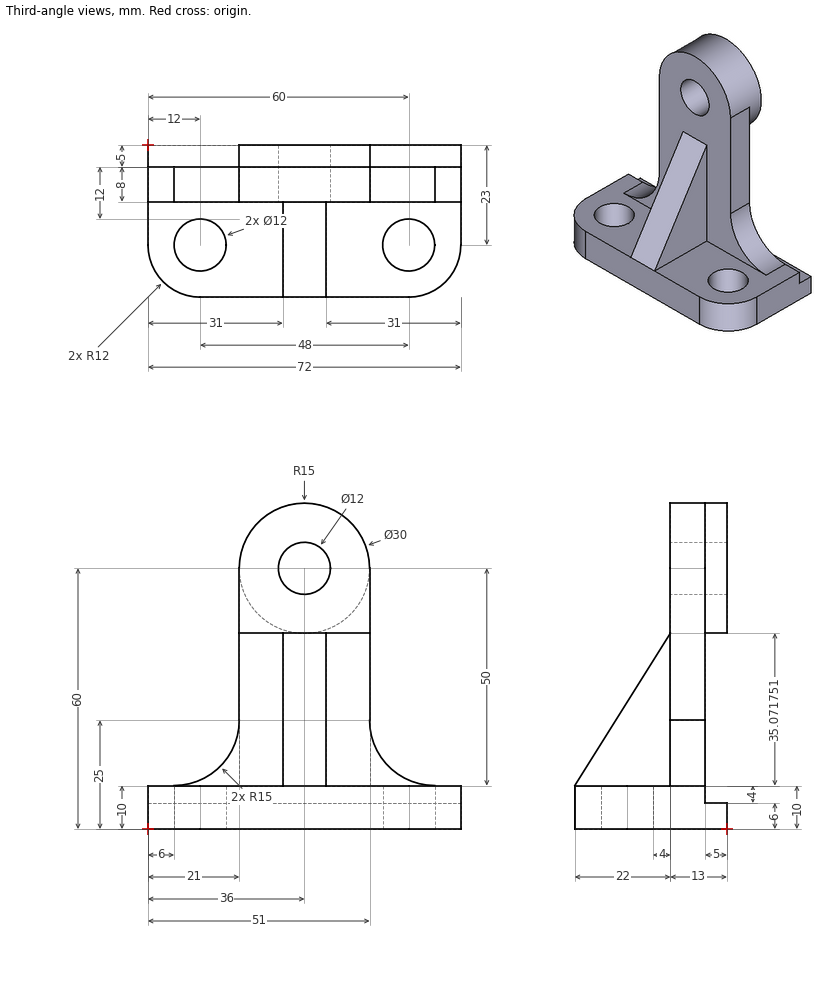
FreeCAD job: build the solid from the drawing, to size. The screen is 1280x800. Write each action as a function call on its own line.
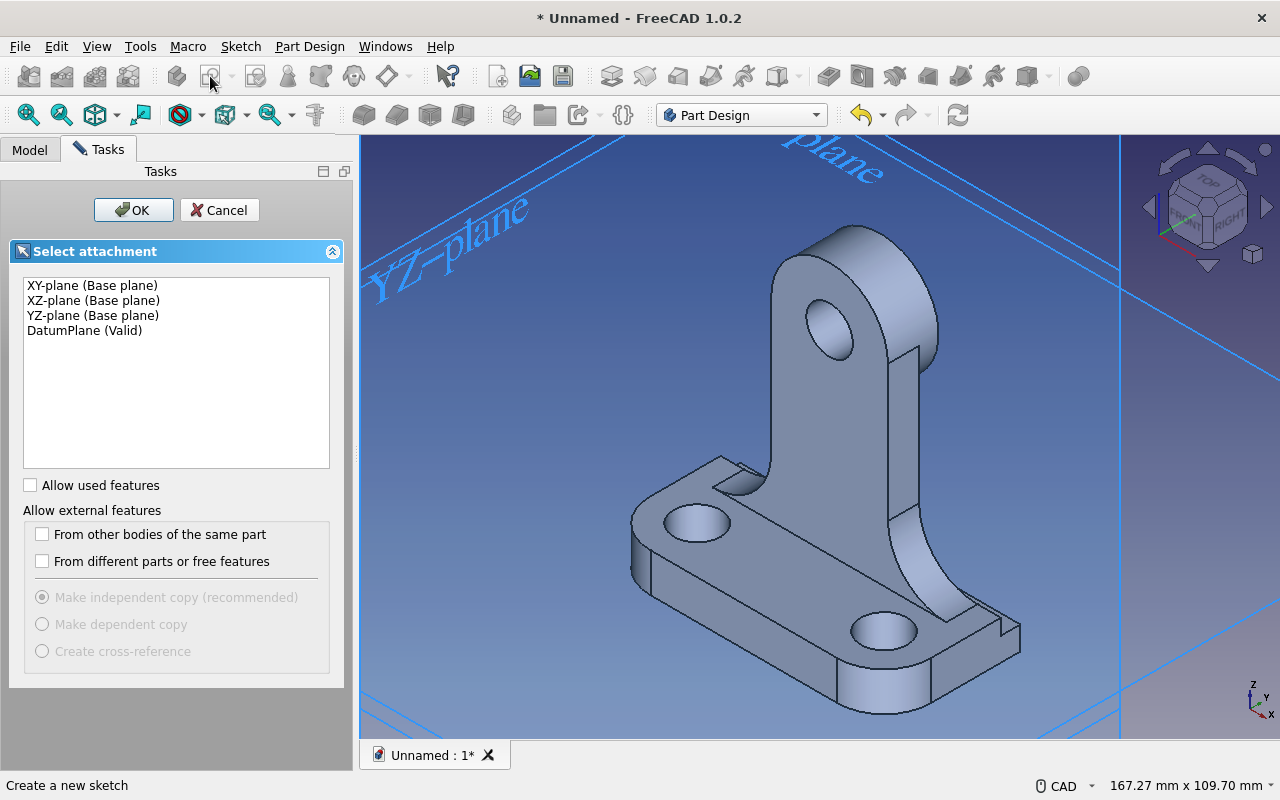
click(84, 316)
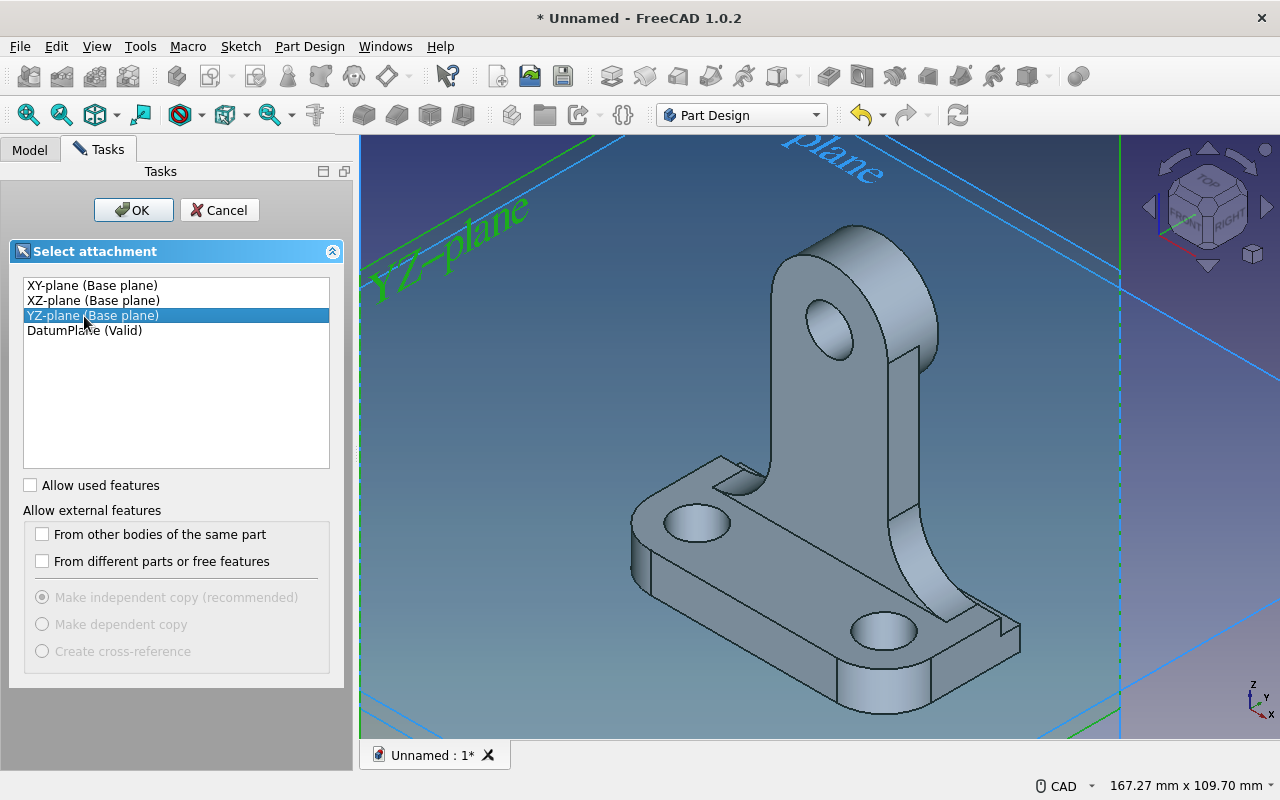
click(134, 210)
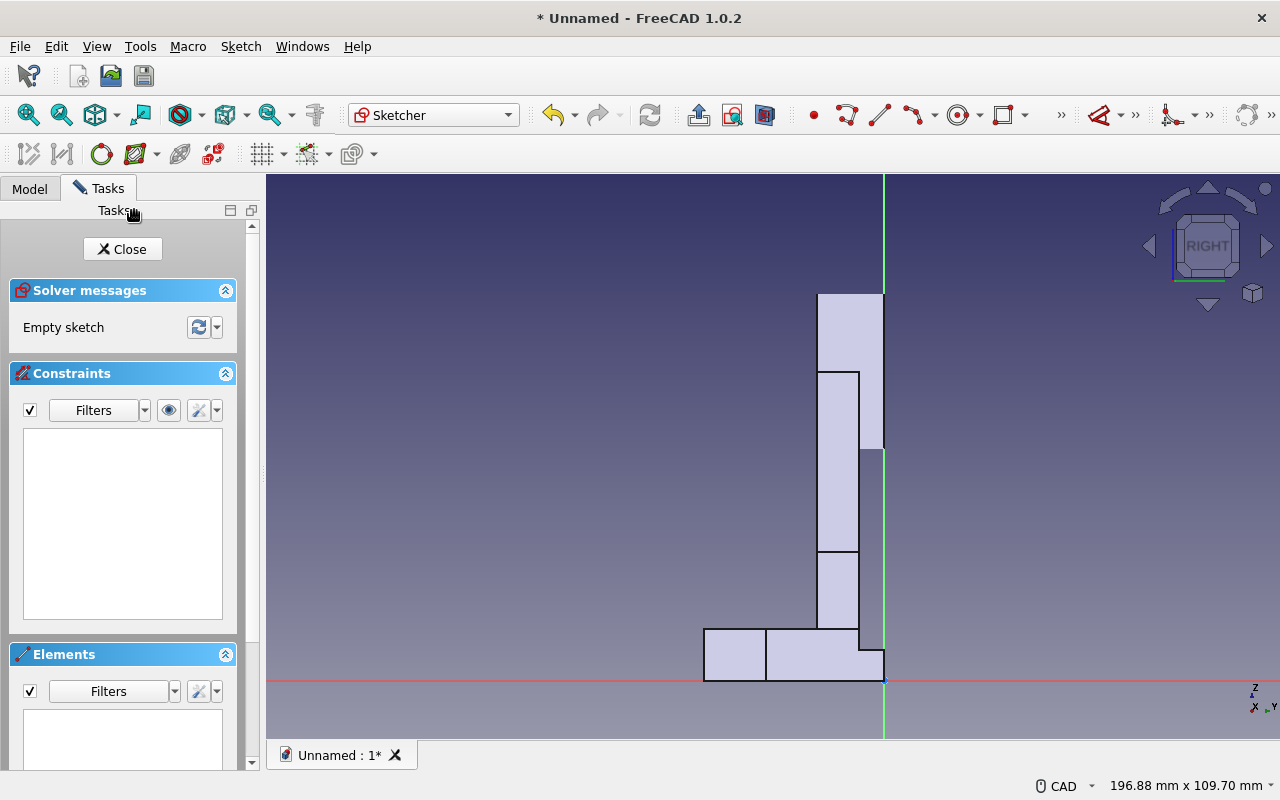
click(765, 116)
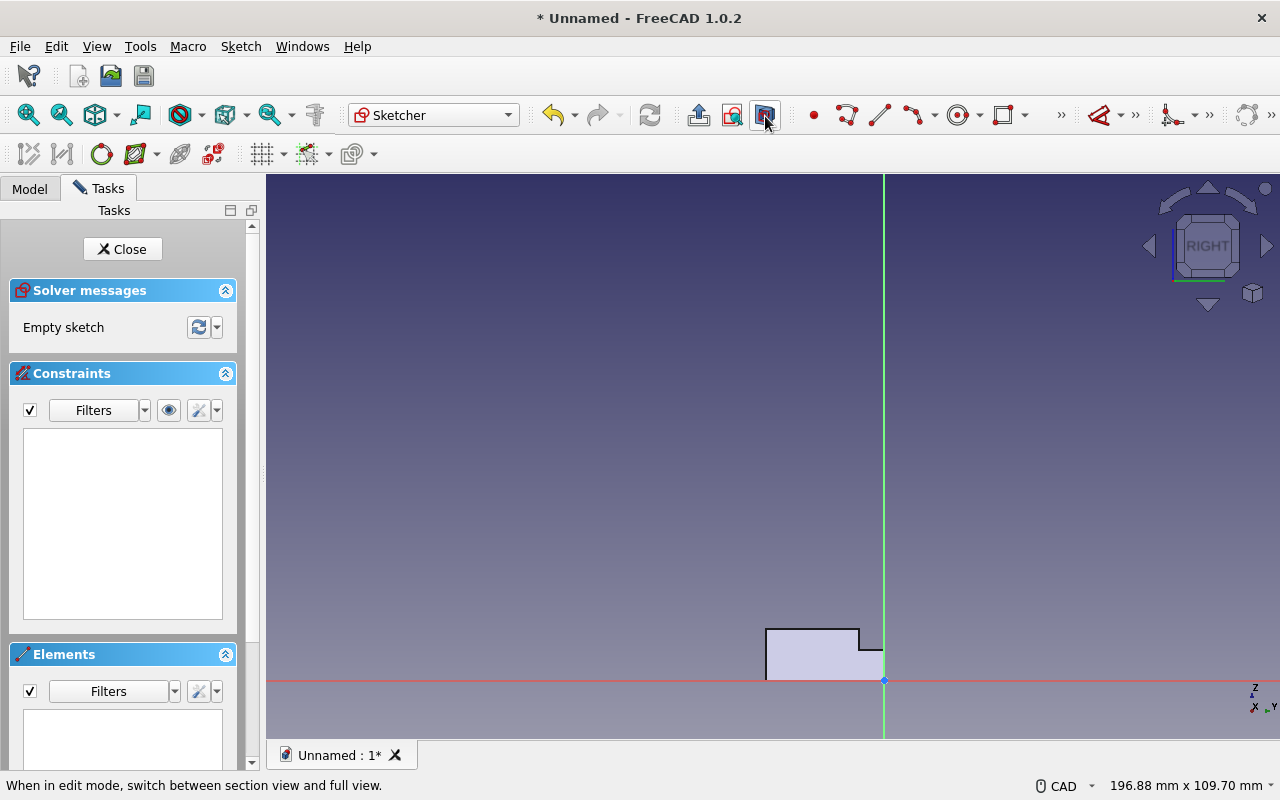
scroll(977, 711, up, 2)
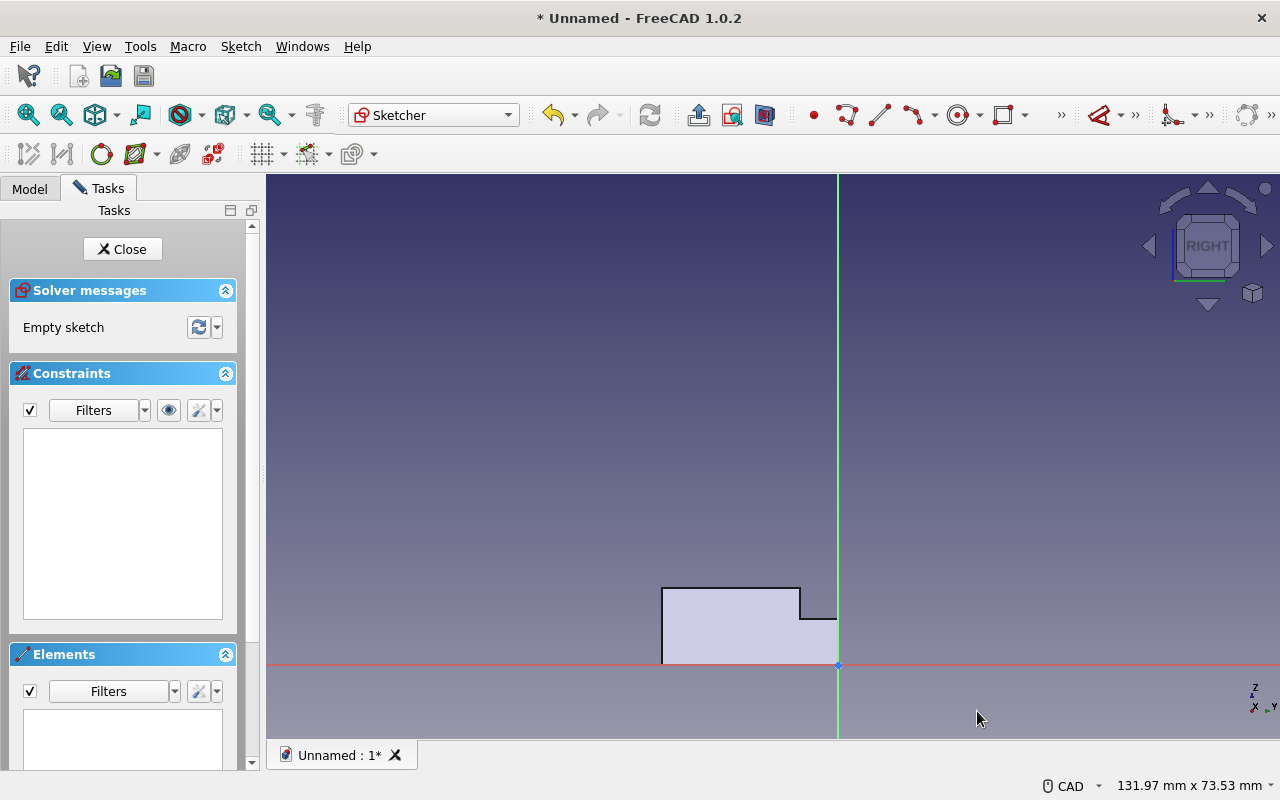
click(847, 116)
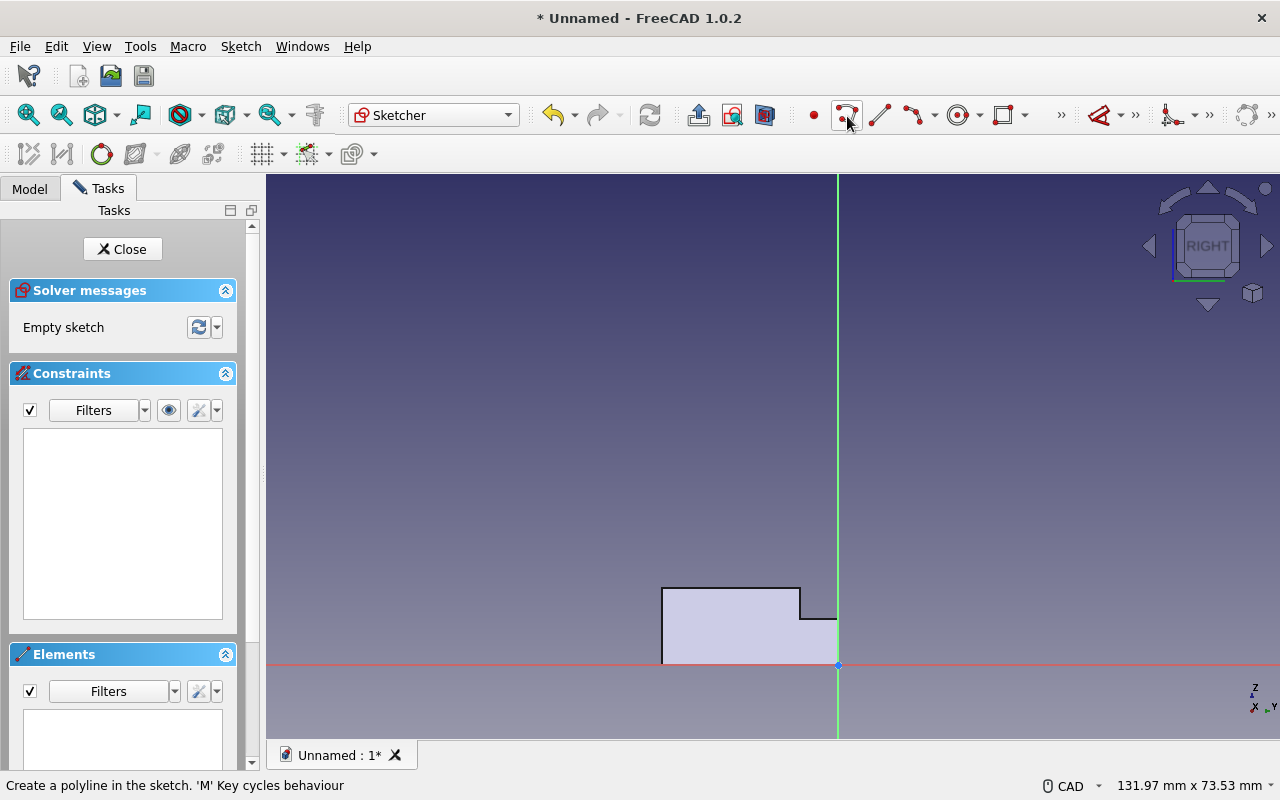
click(739, 588)
click(569, 588)
click(739, 319)
click(739, 589)
key(Escape)
key(Escape)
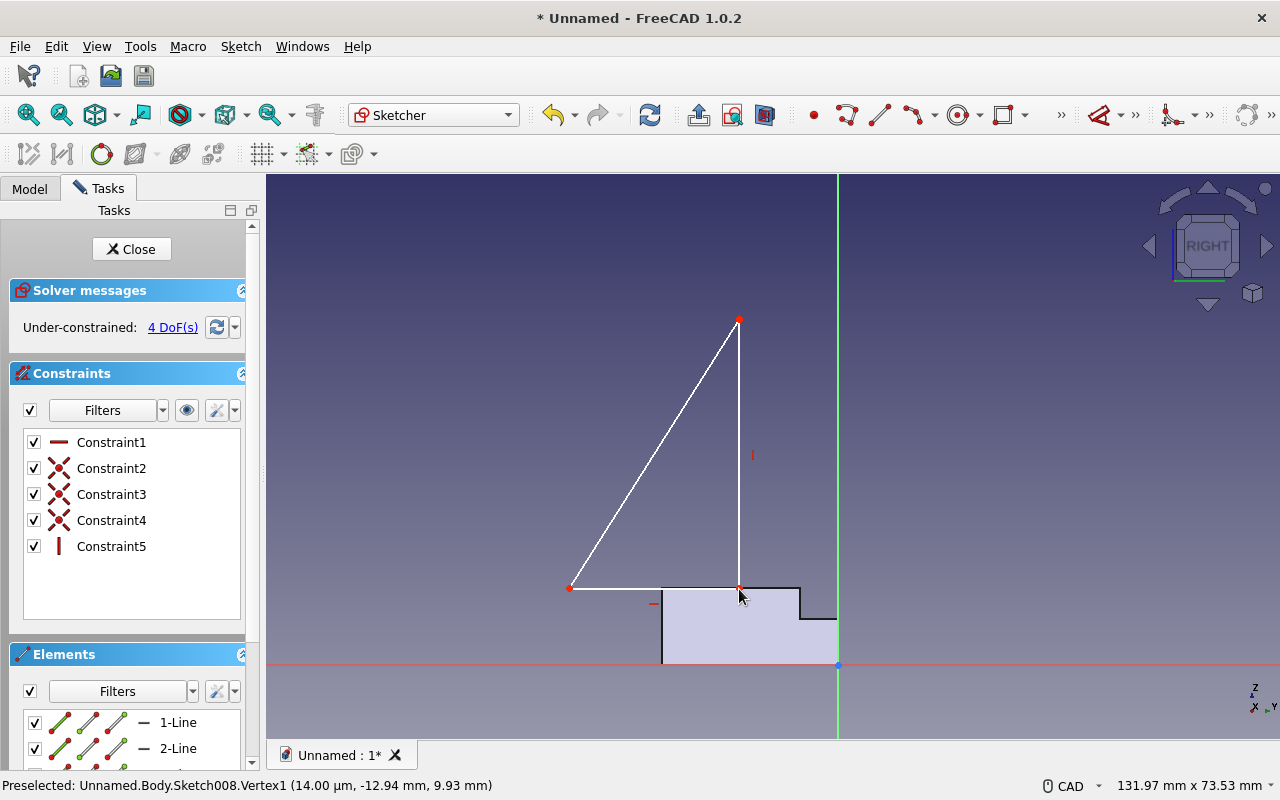
click(1098, 116)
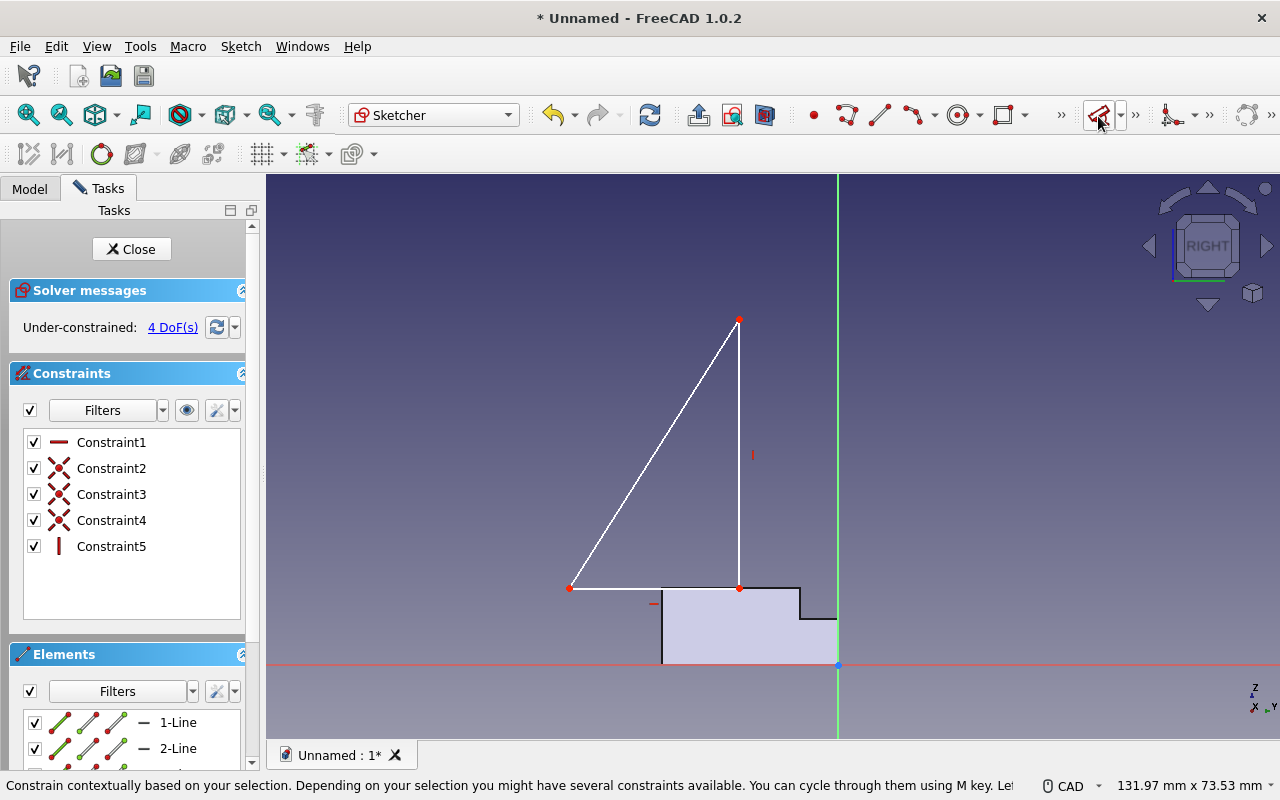
click(688, 589)
click(654, 623)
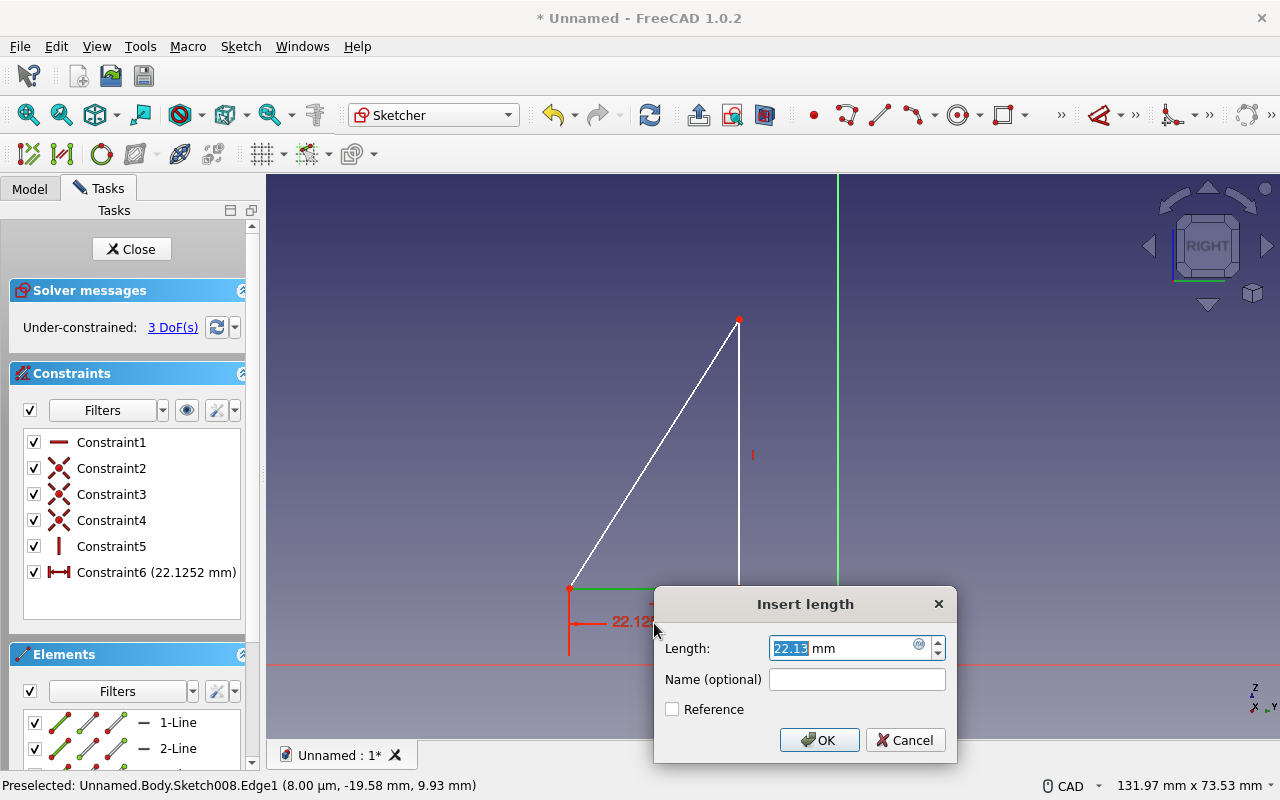
text(22)
key(Return)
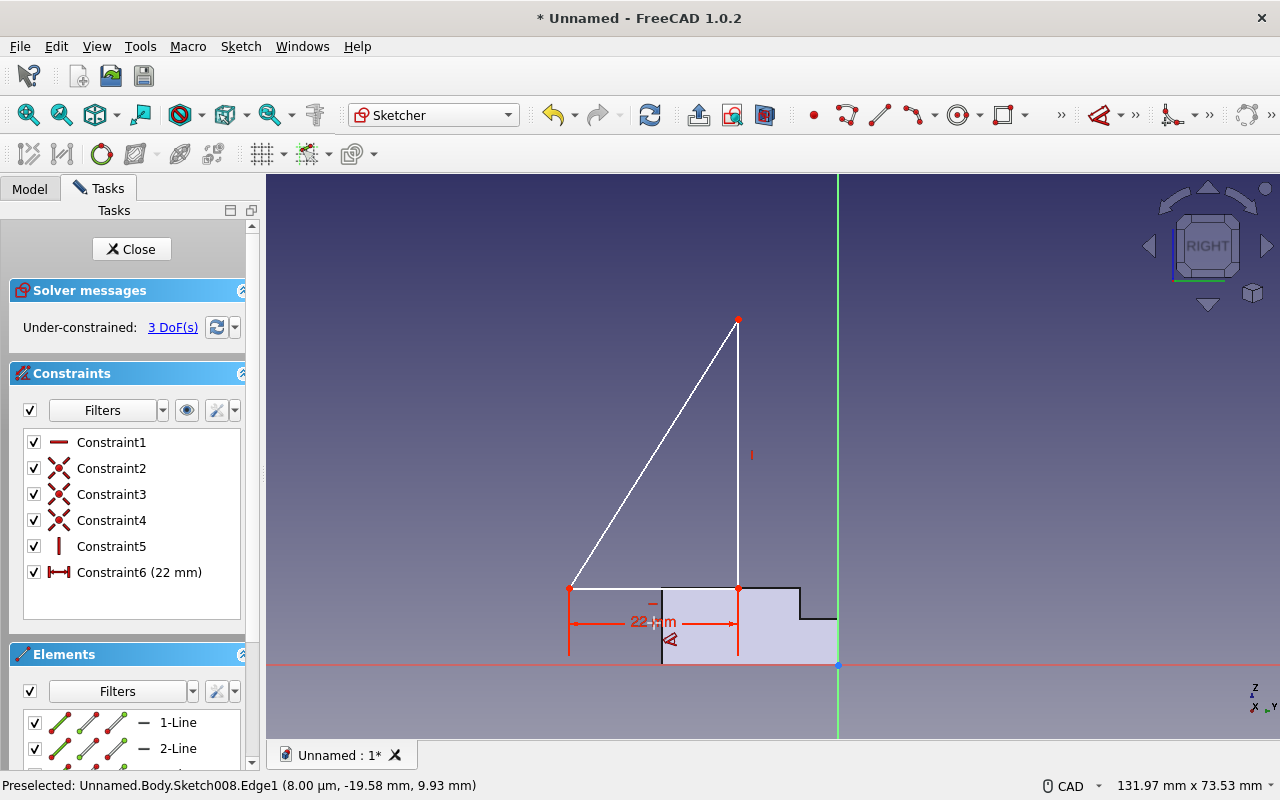
click(738, 589)
click(788, 699)